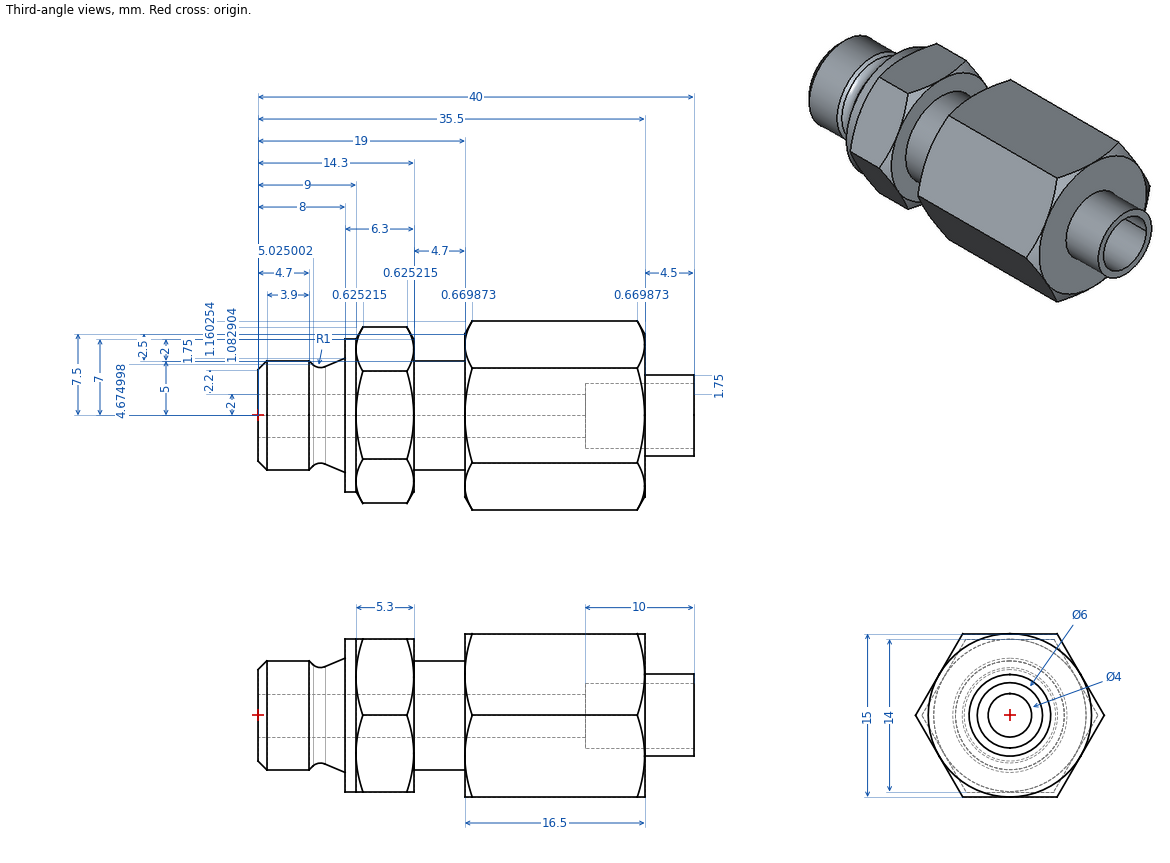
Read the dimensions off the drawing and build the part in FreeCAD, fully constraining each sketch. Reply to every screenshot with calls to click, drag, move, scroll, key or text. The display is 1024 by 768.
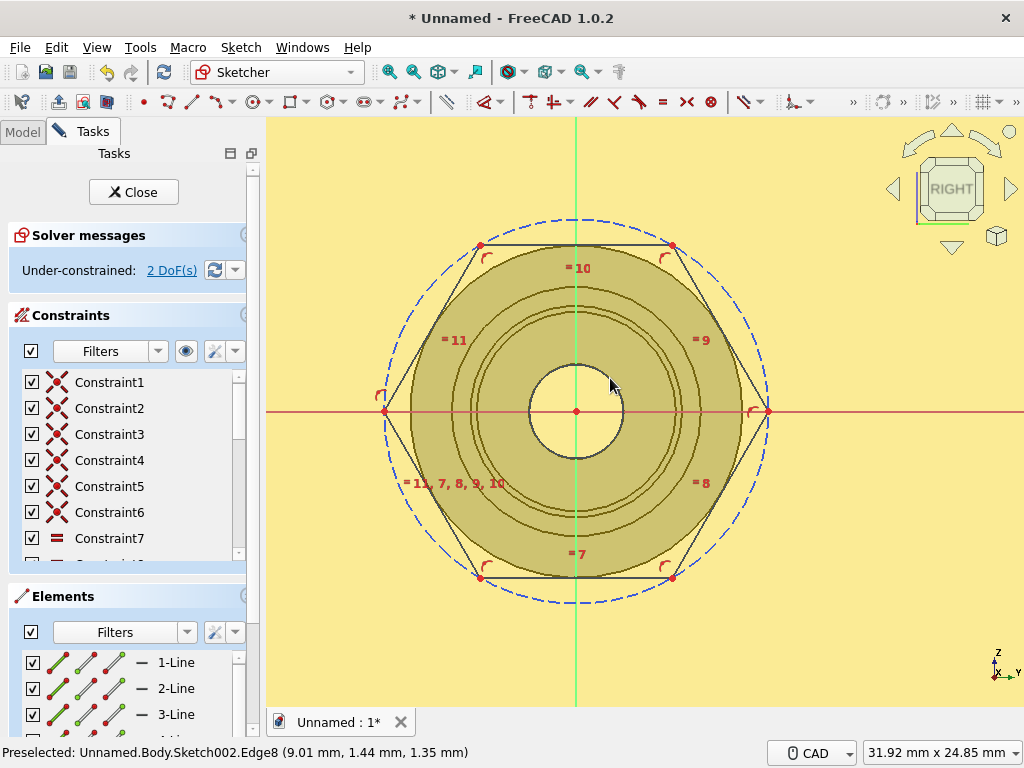
key(d)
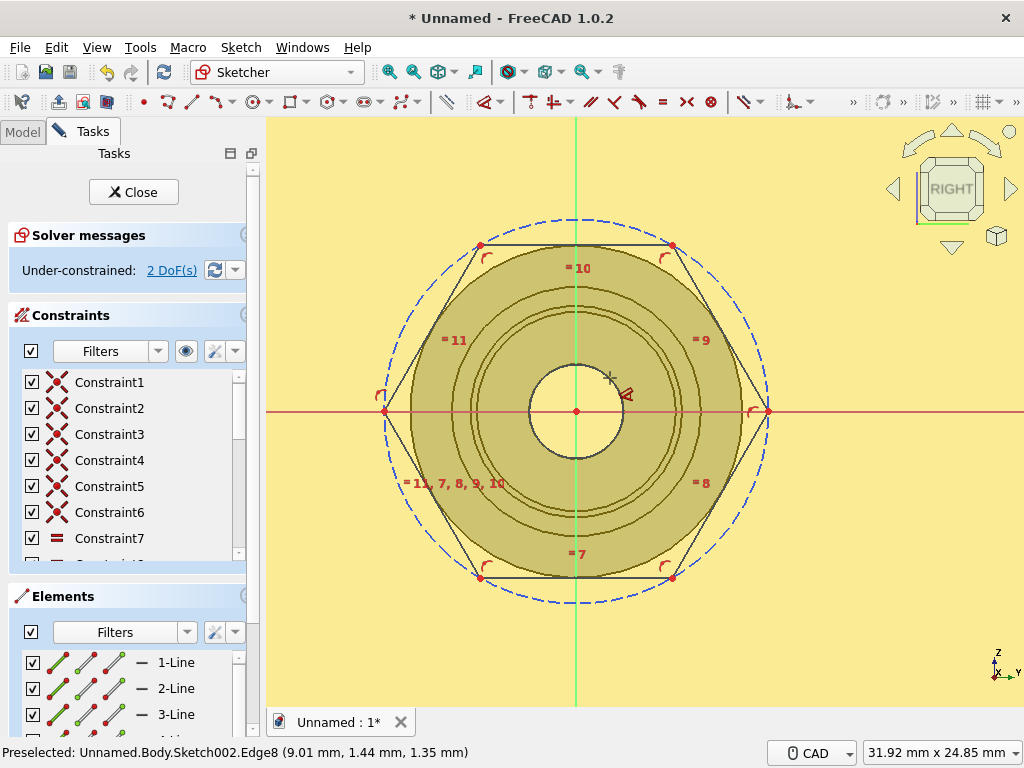
click(609, 378)
click(631, 355)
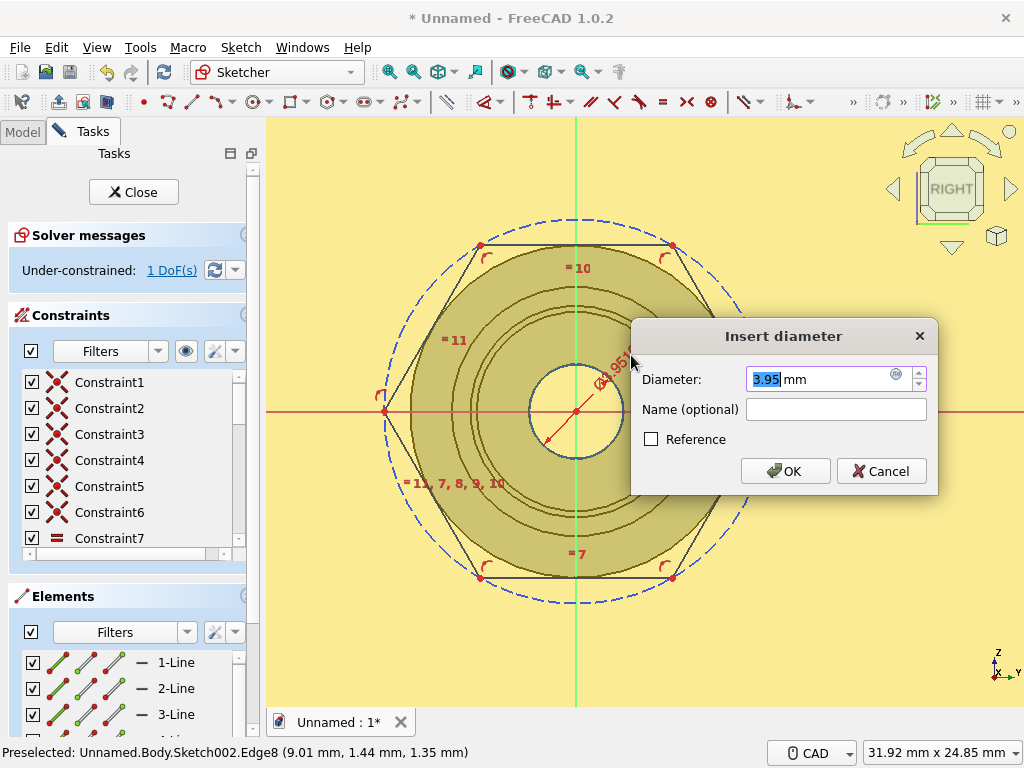
text(4)
key(Return)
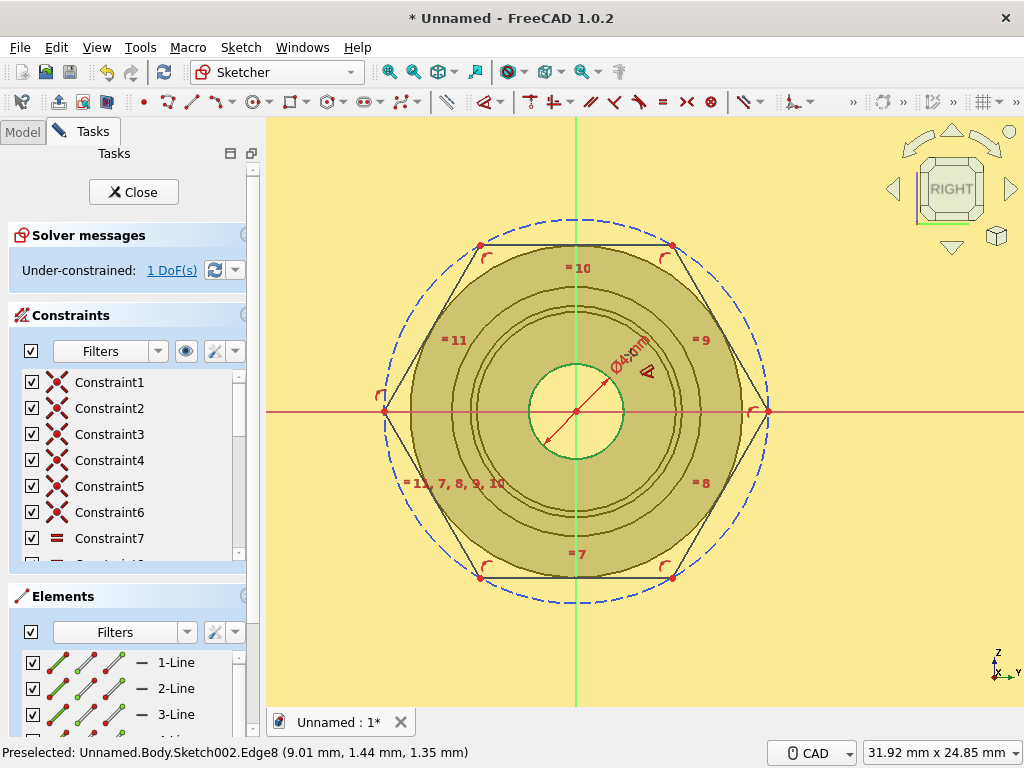
click(480, 578)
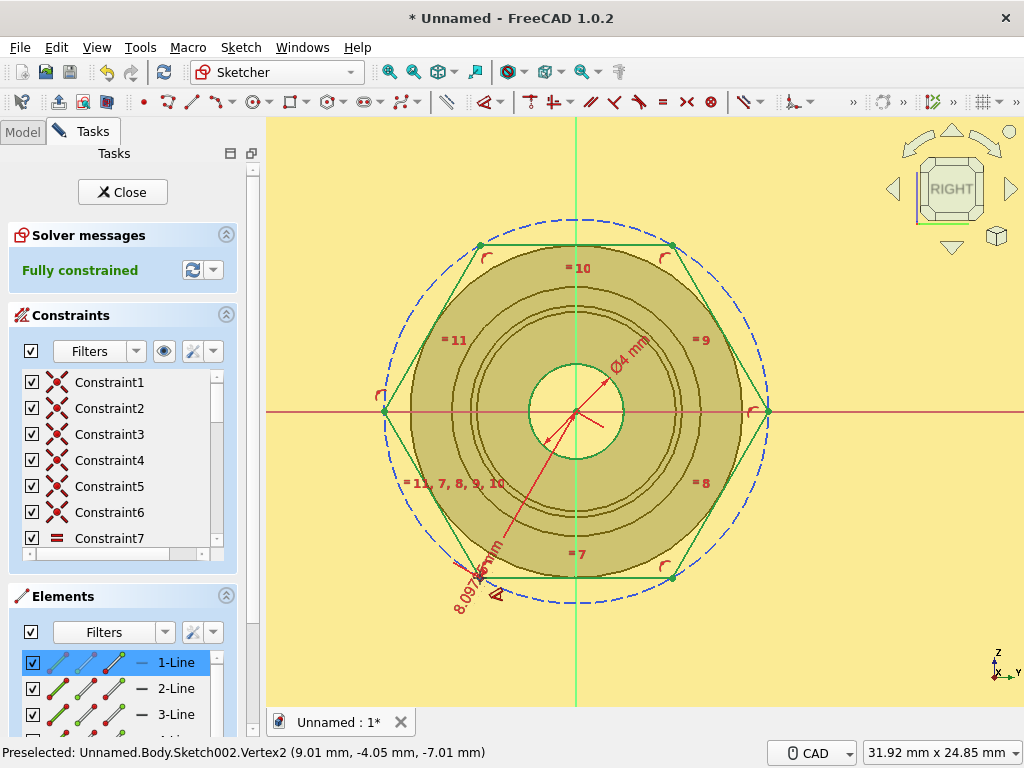
click(672, 245)
click(706, 335)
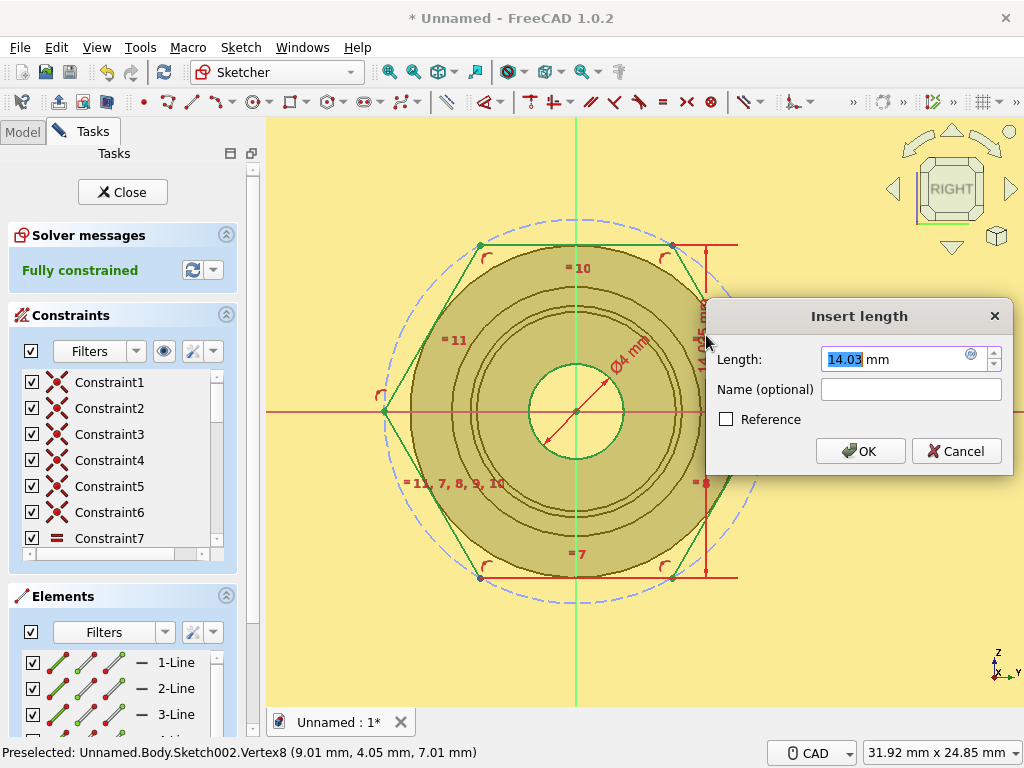
text(14)
key(Return)
key(Escape)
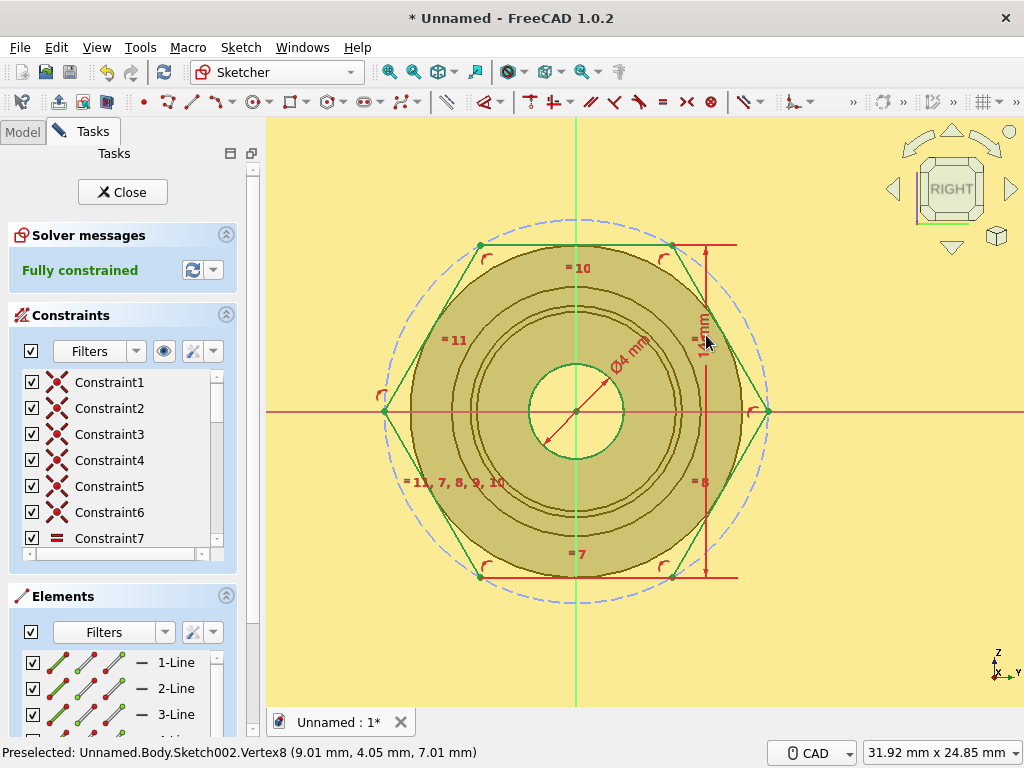
click(123, 192)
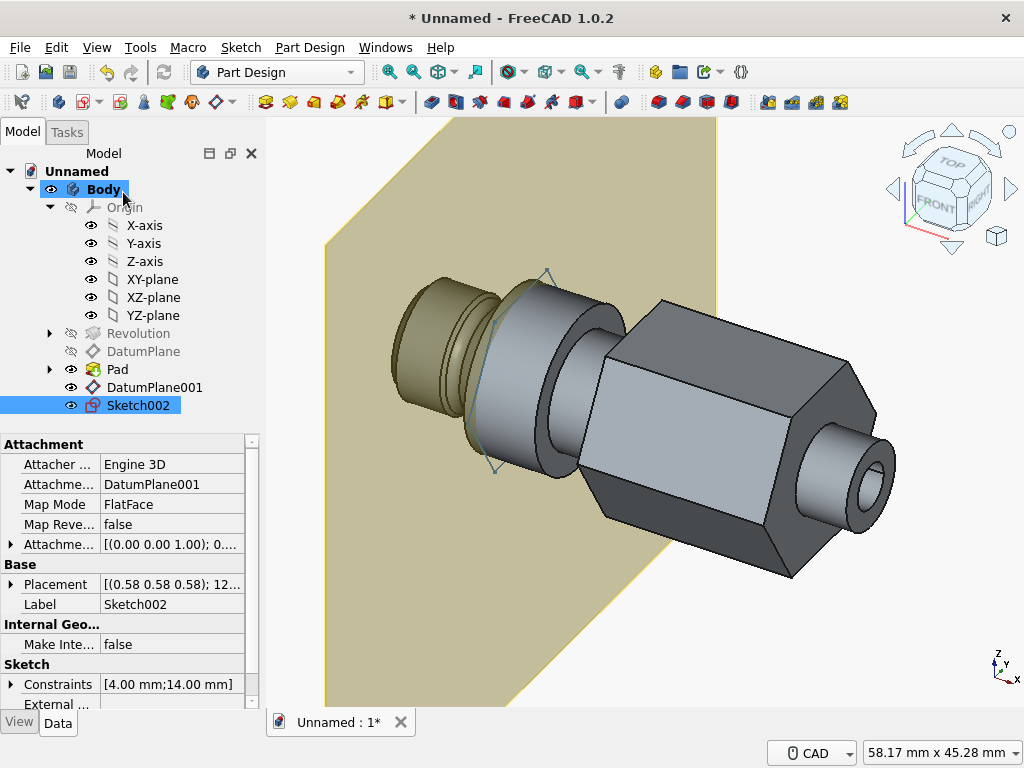
click(266, 102)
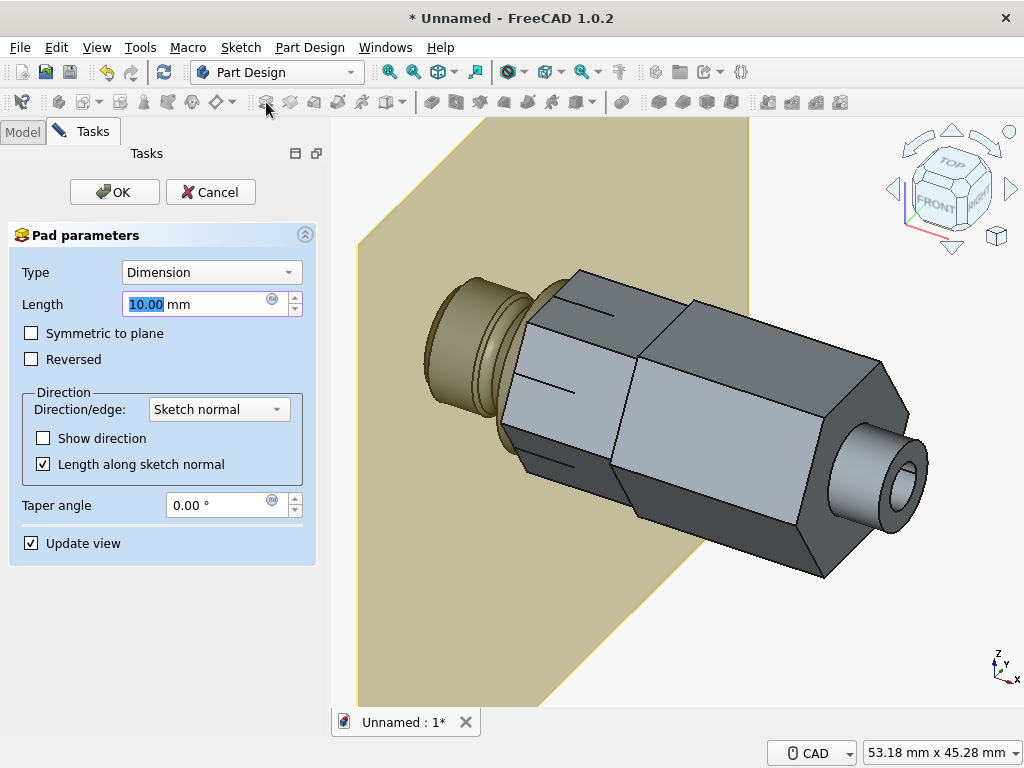
text(5.3)
key(Tab)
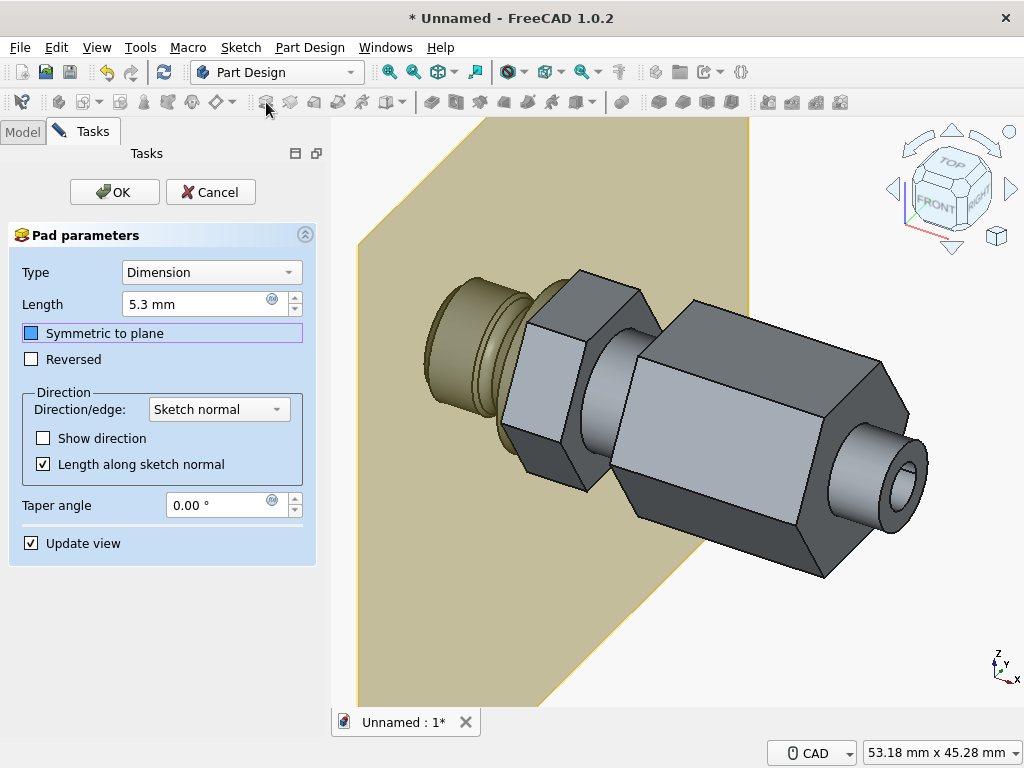
click(115, 192)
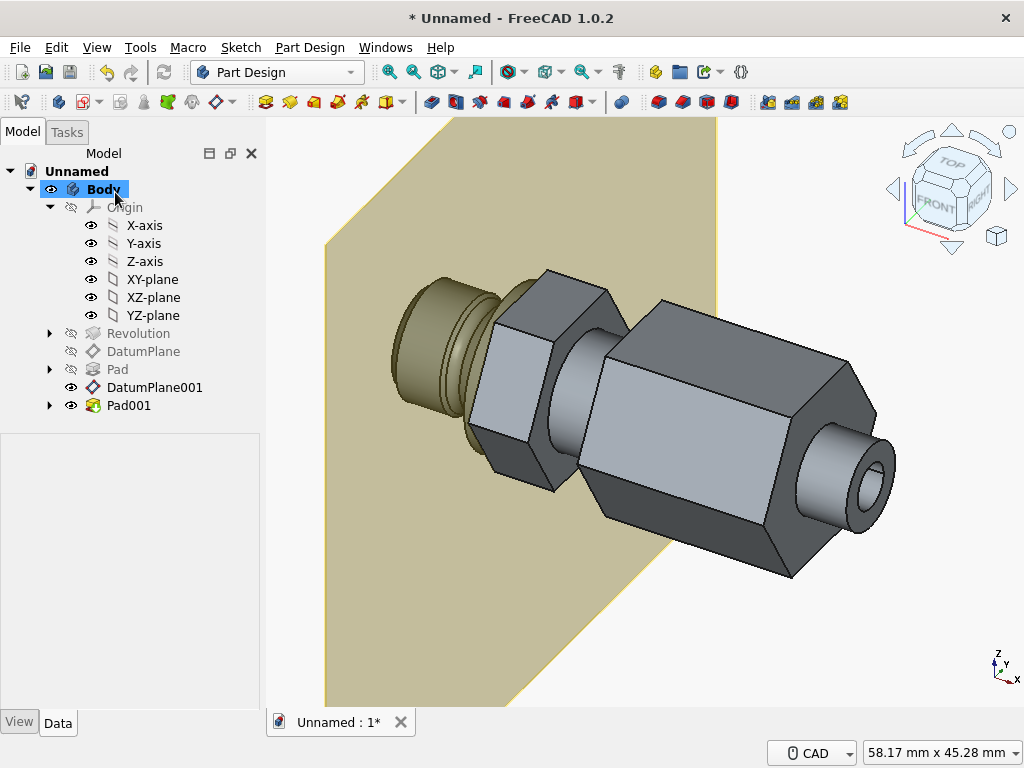
click(116, 387)
key(space)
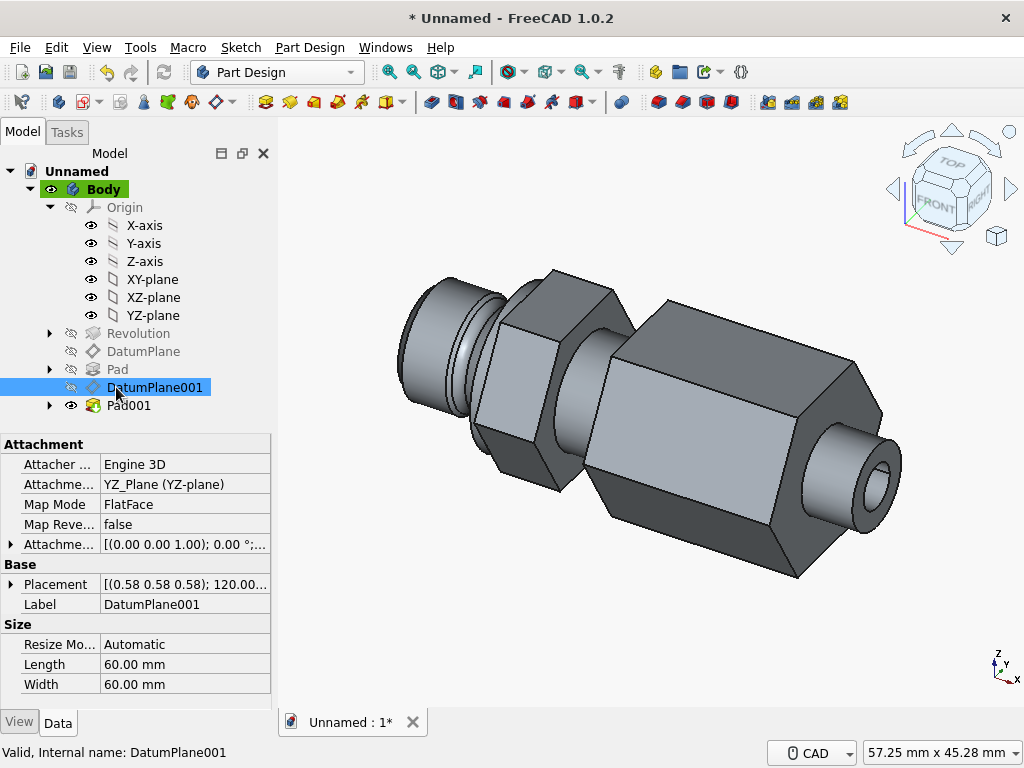
click(318, 667)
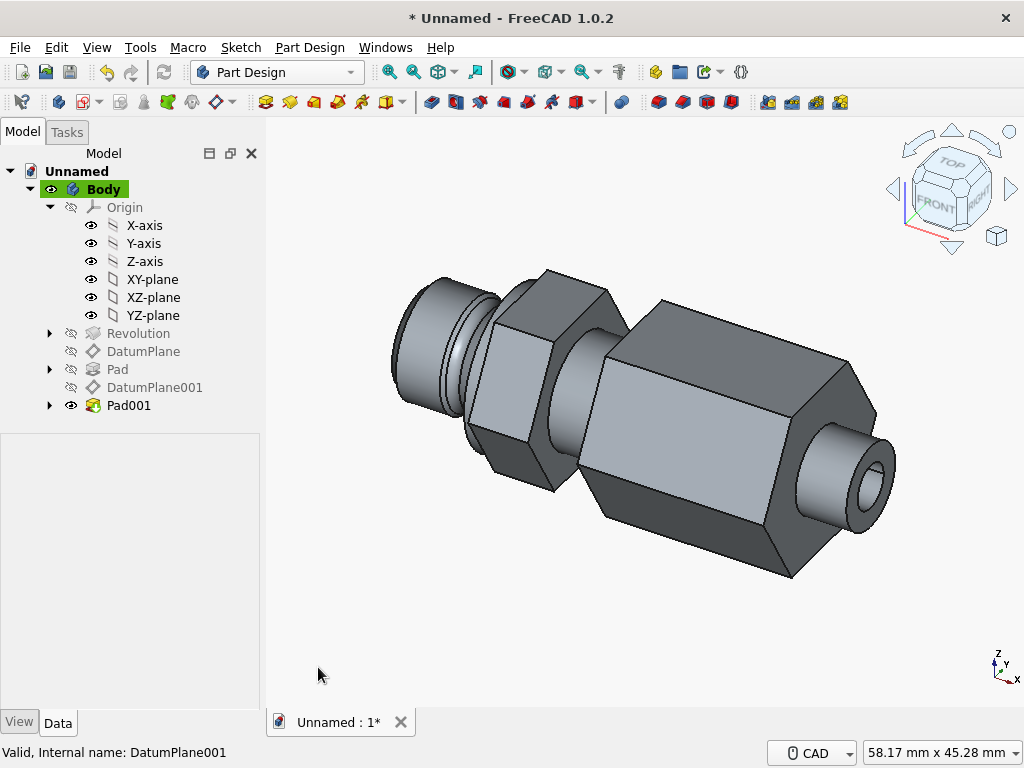
click(84, 102)